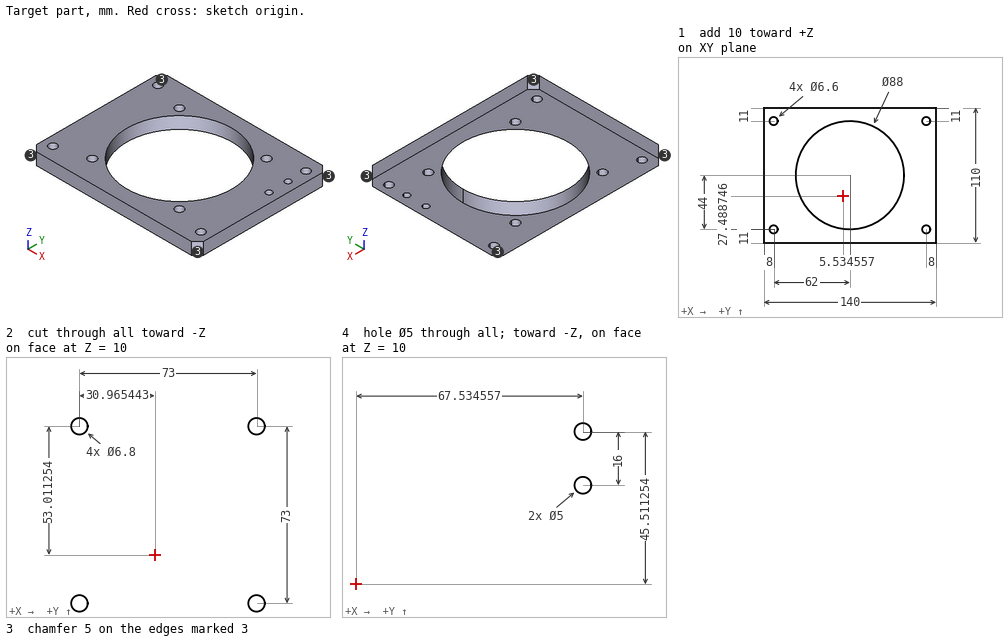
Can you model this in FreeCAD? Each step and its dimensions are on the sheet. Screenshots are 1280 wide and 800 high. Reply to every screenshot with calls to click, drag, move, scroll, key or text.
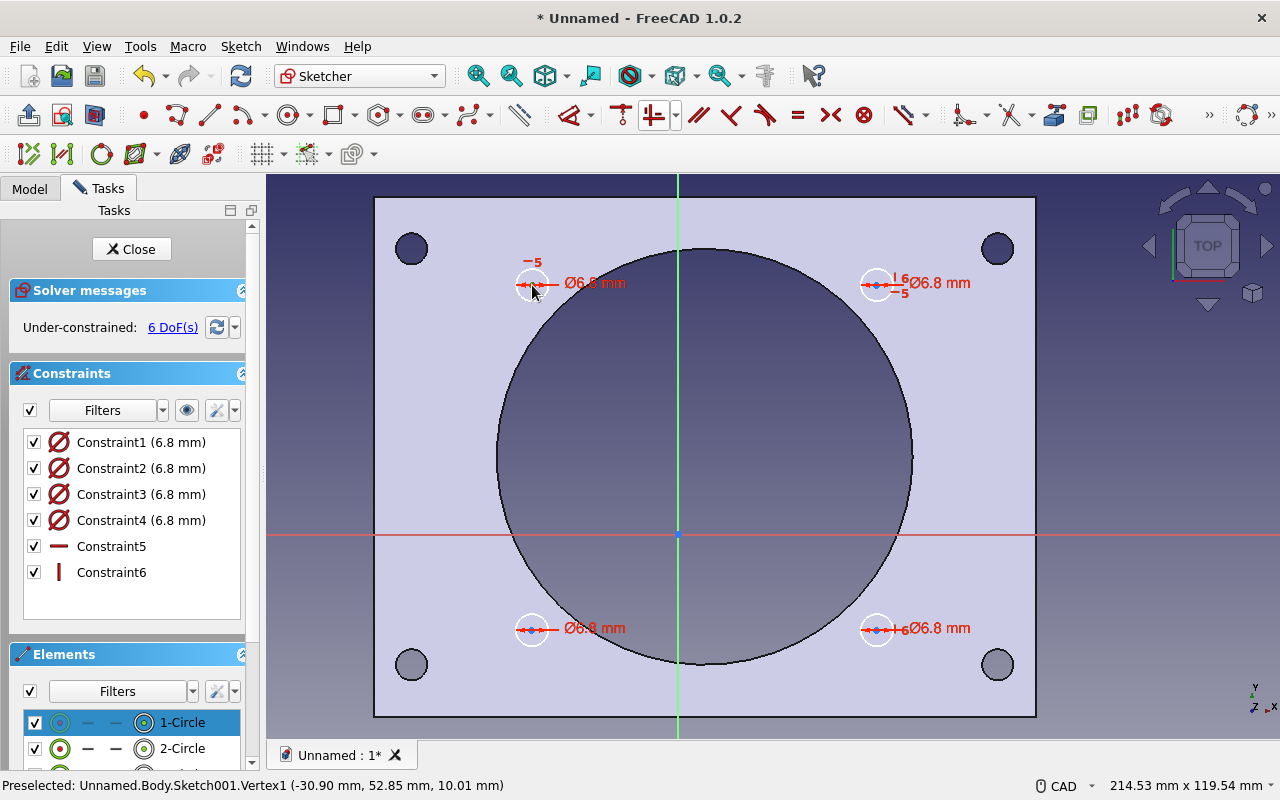
click(532, 630)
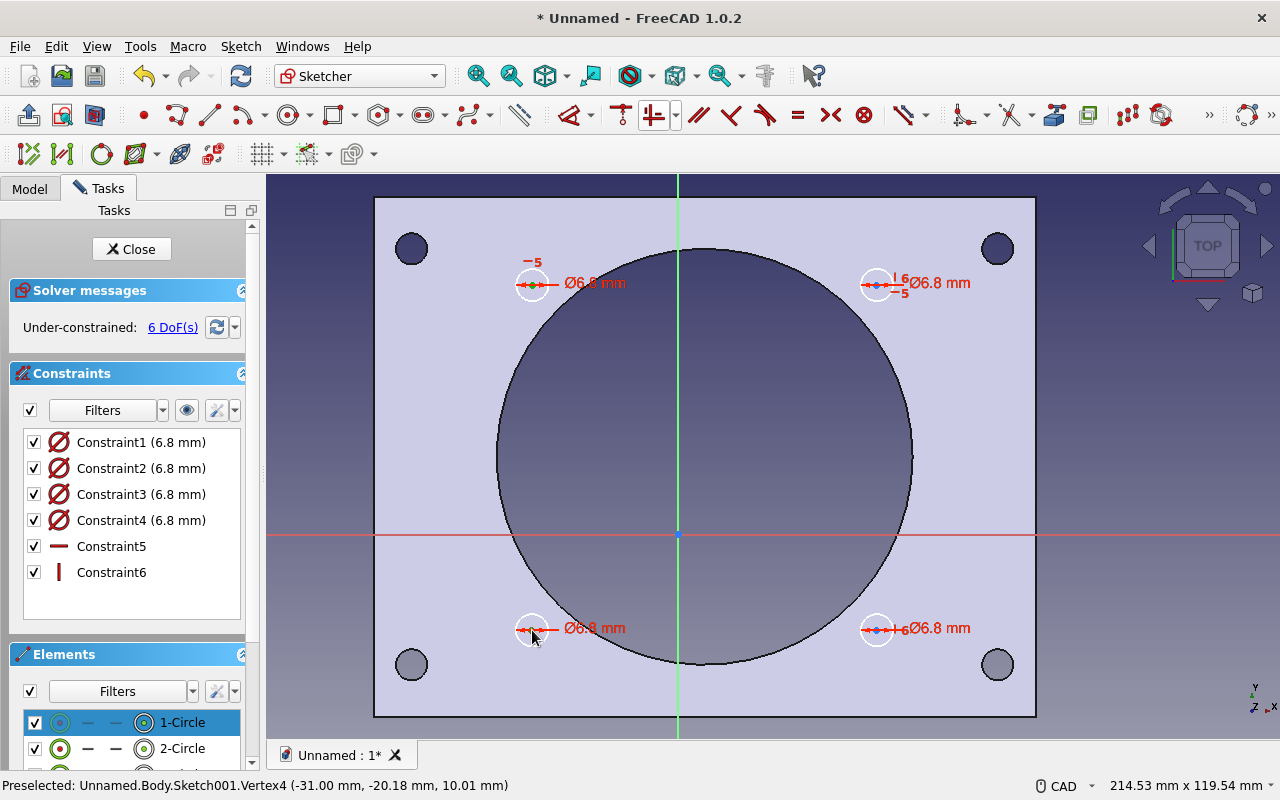
click(676, 116)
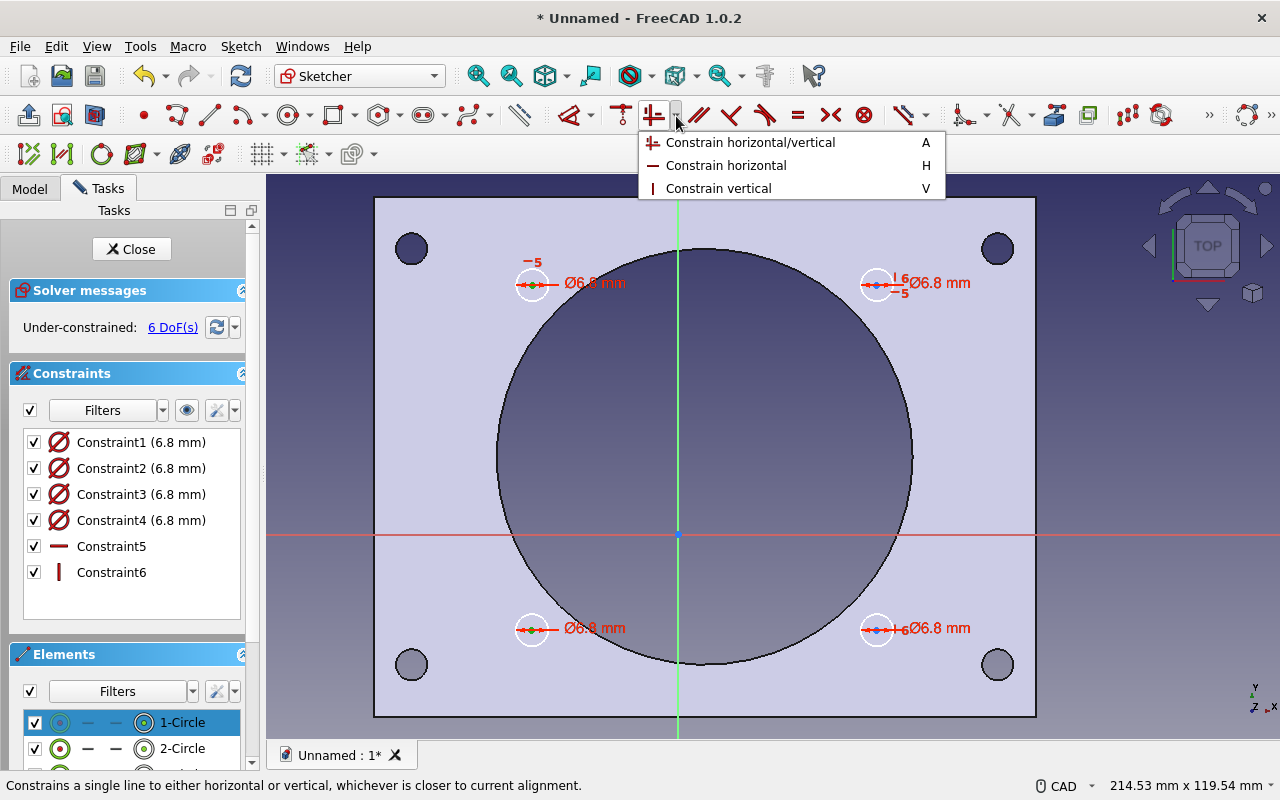
click(792, 188)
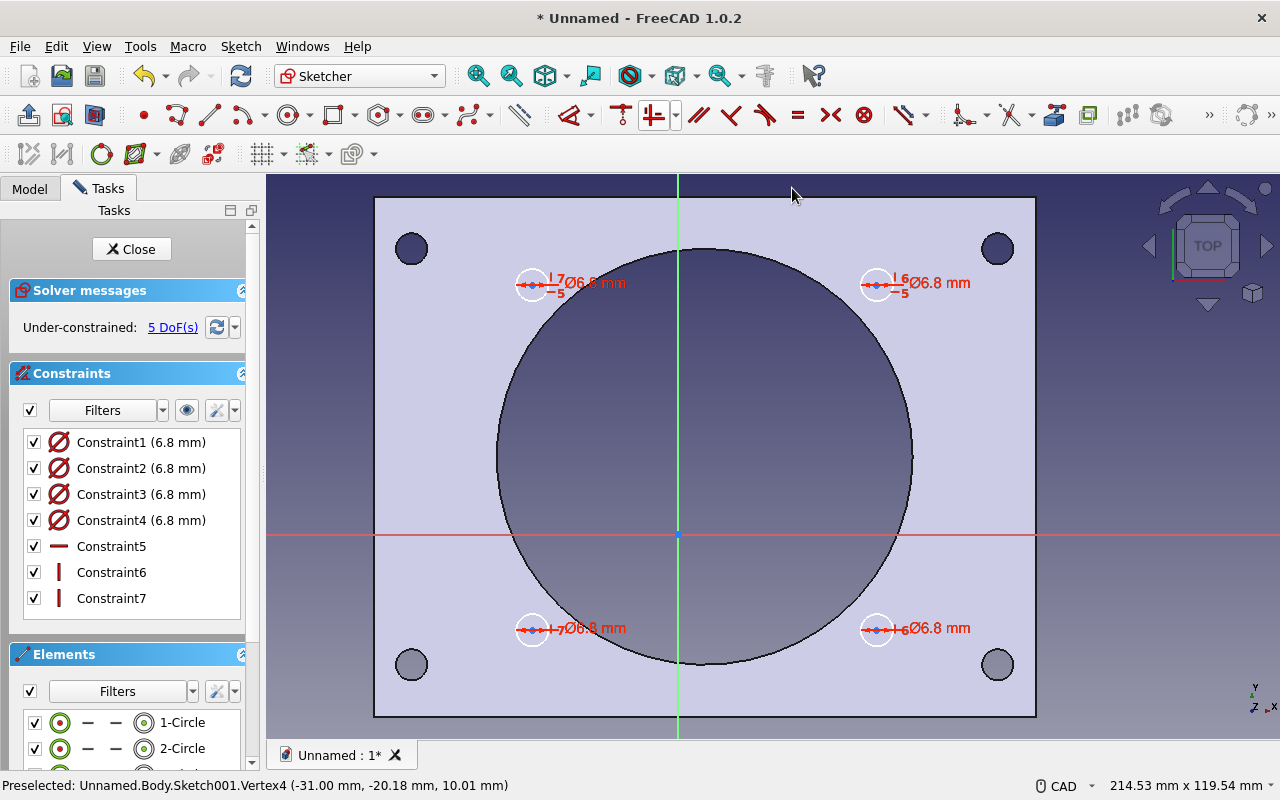
click(877, 630)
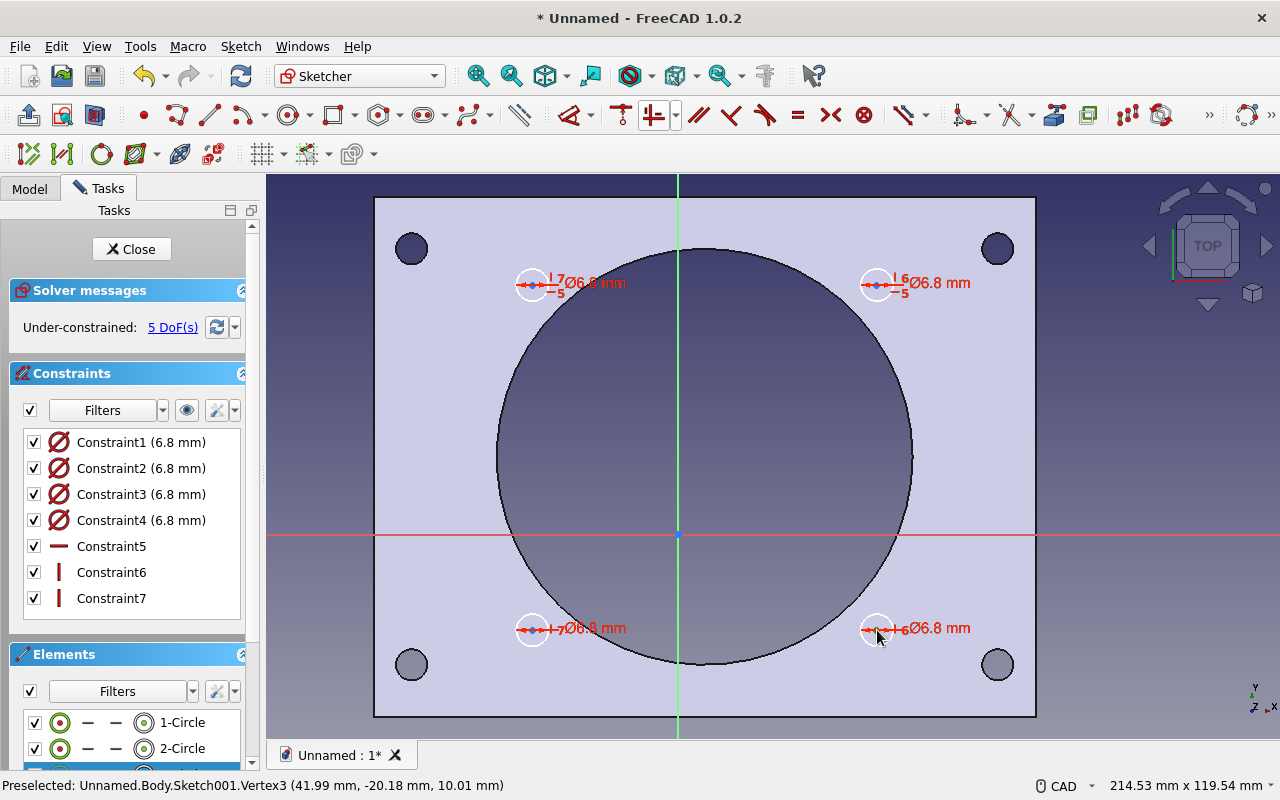
click(532, 630)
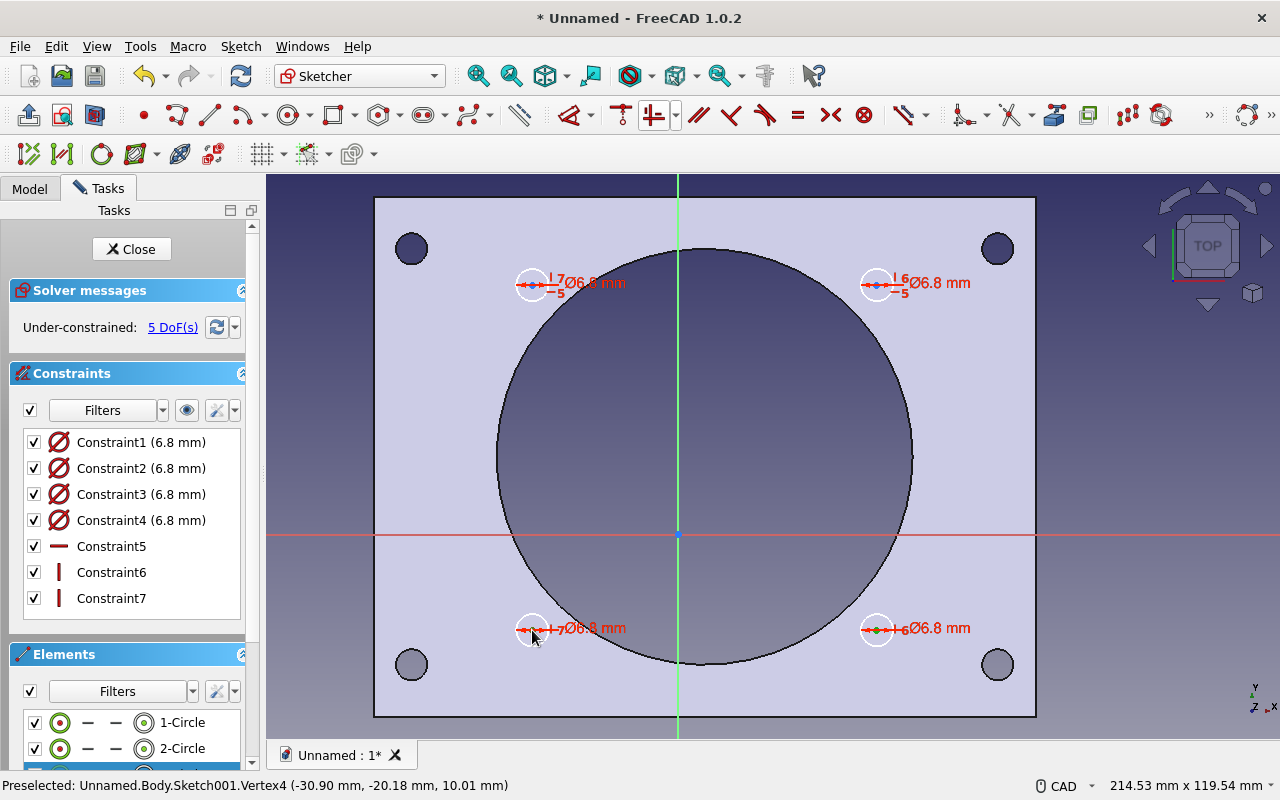
click(676, 116)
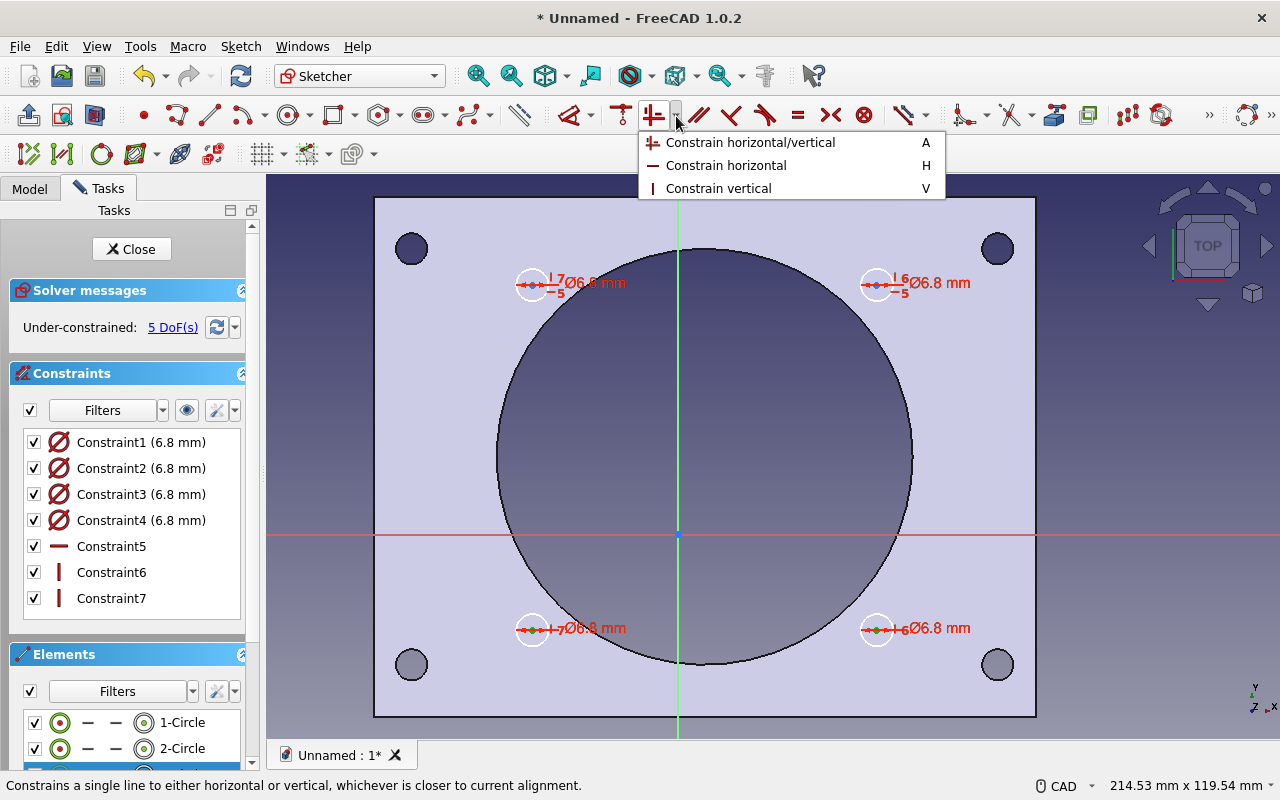
click(792, 166)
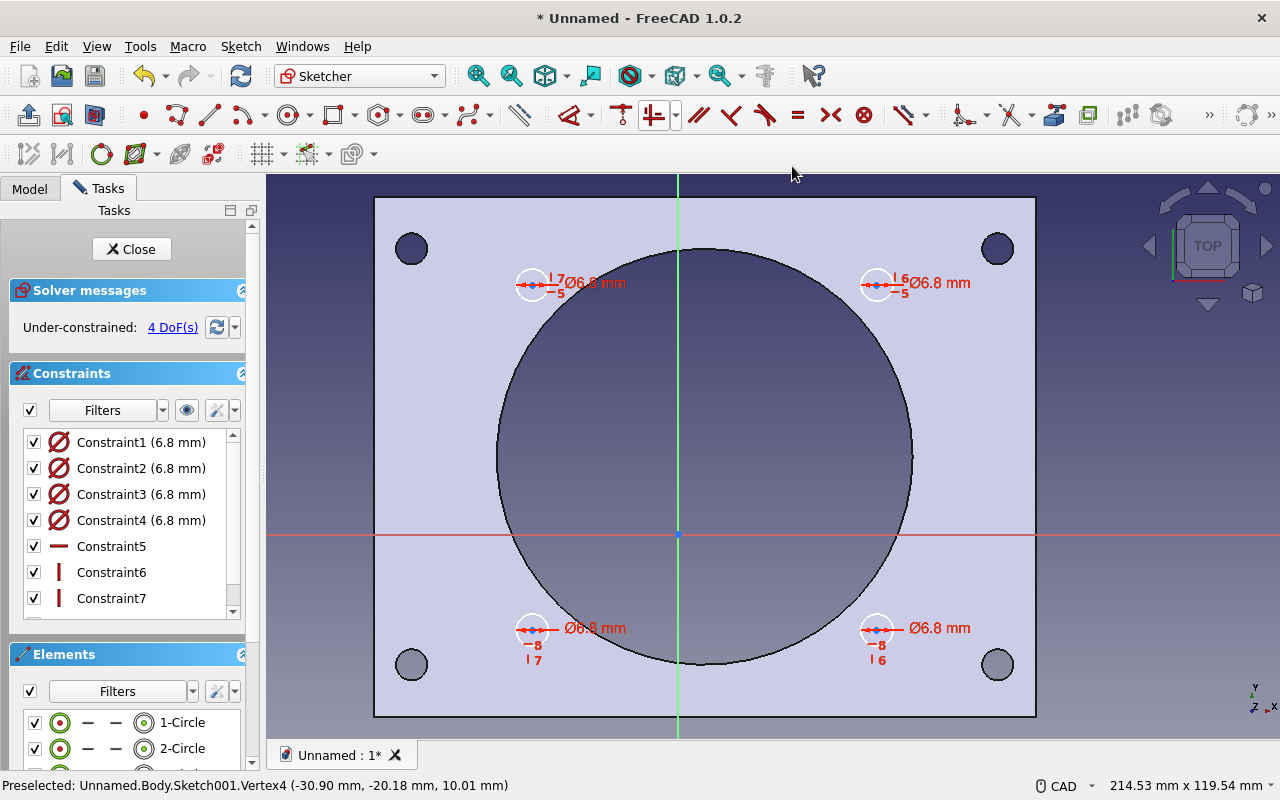
click(568, 116)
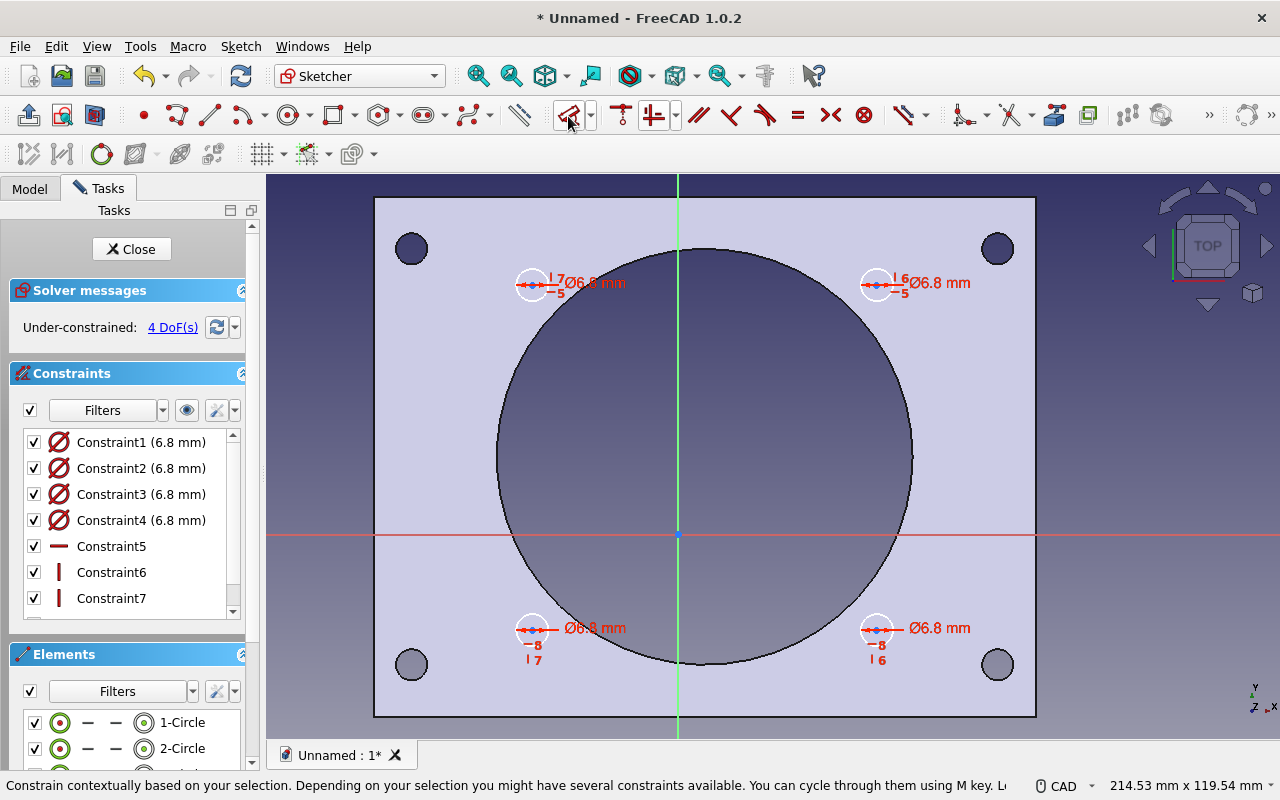
click(532, 285)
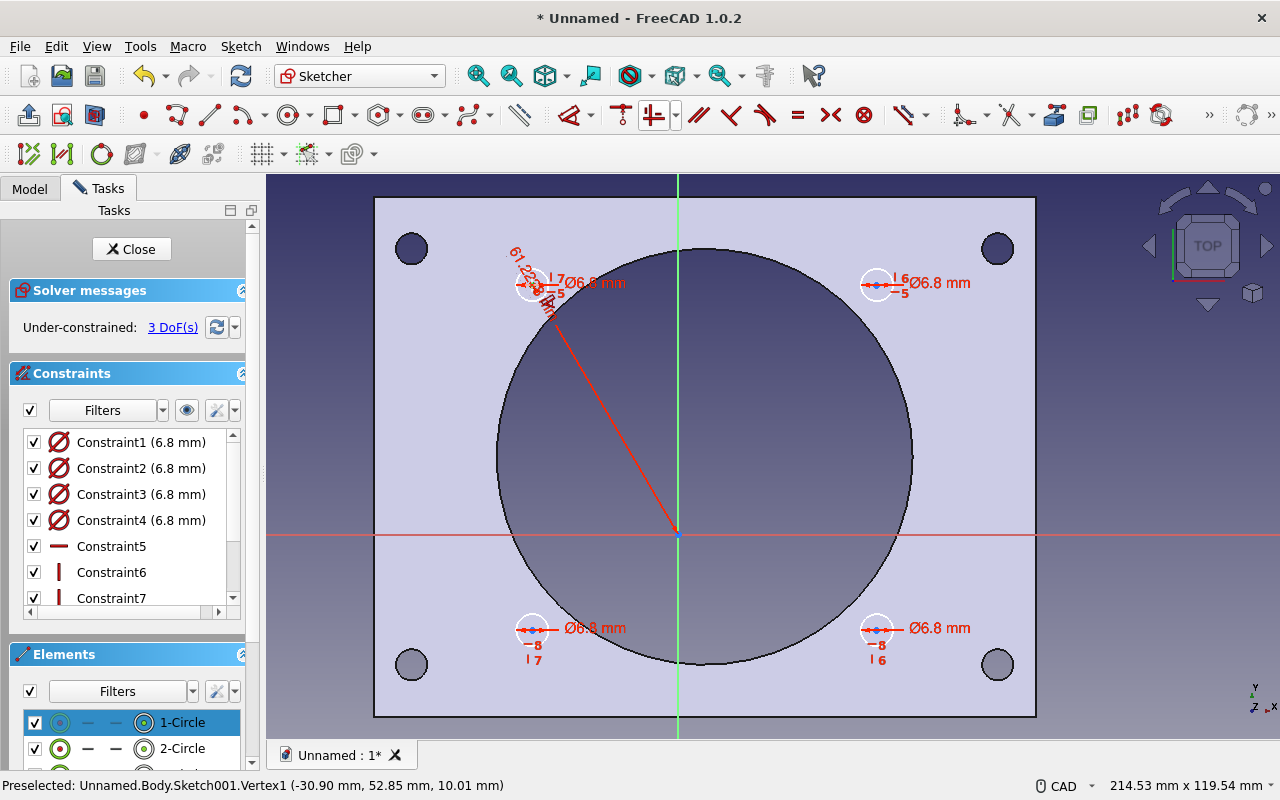
click(877, 285)
click(705, 251)